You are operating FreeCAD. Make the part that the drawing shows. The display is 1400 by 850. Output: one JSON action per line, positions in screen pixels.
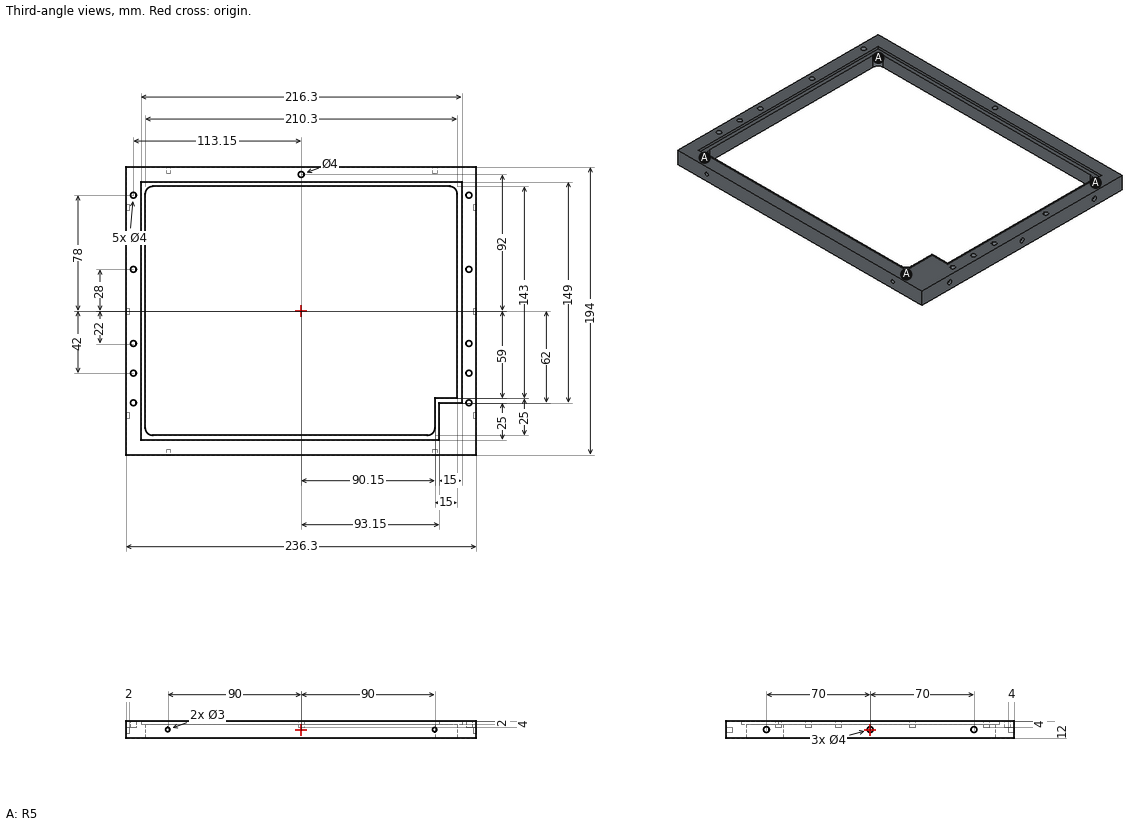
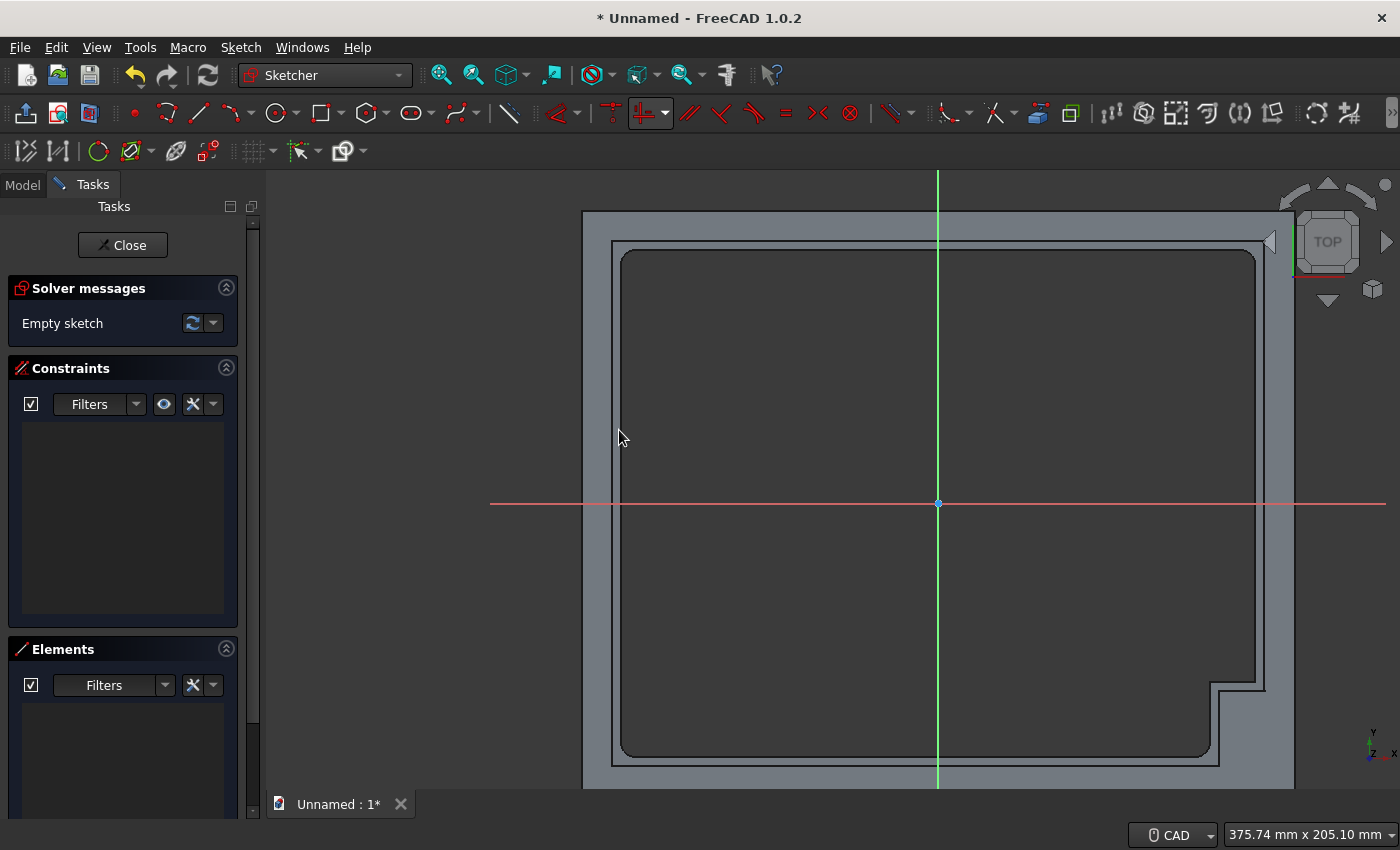
{"action": "left_click", "coordinate": [276, 114]}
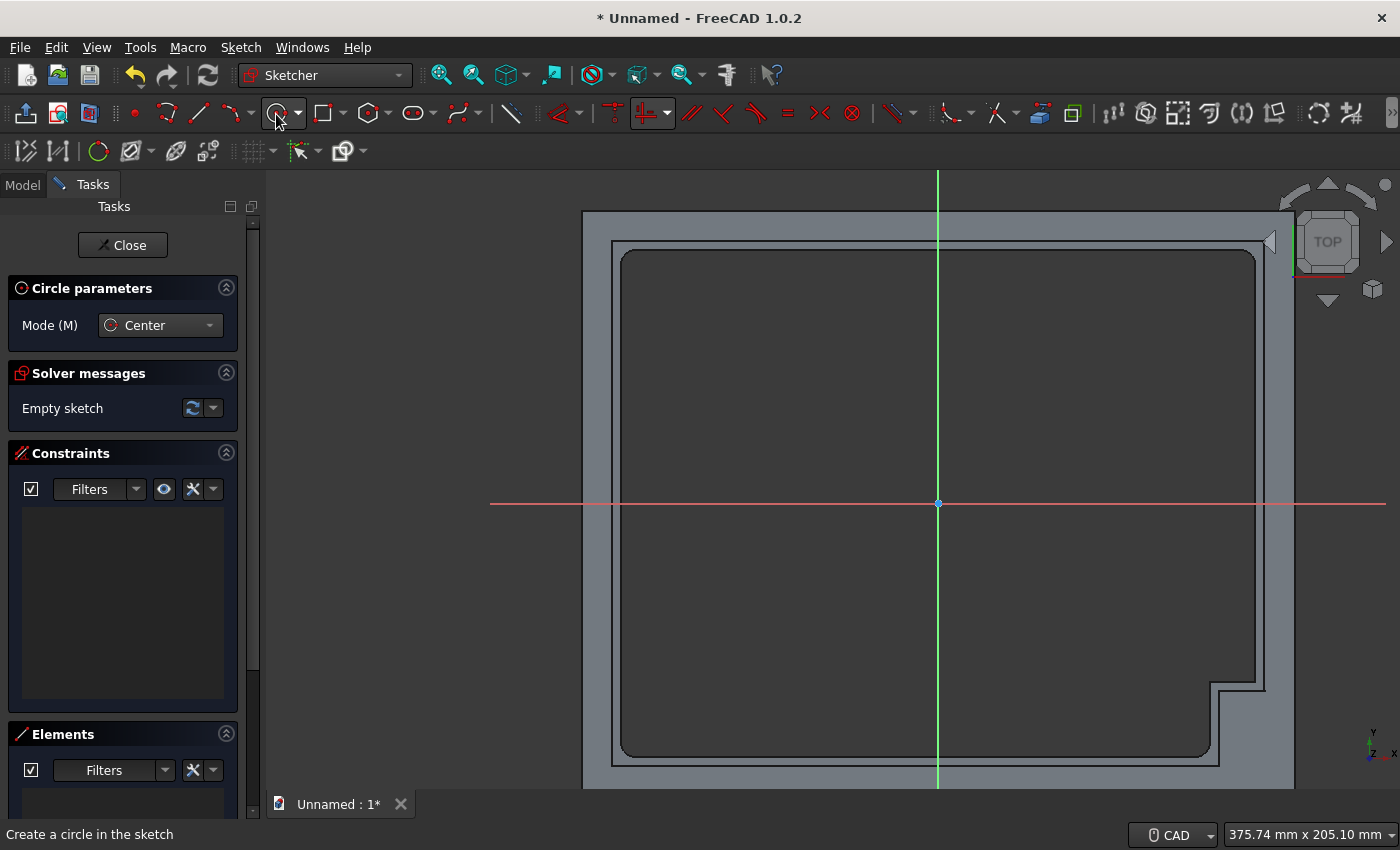
{"action": "scroll", "coordinate": [597, 268], "scroll_direction": "up", "scroll_amount": 7}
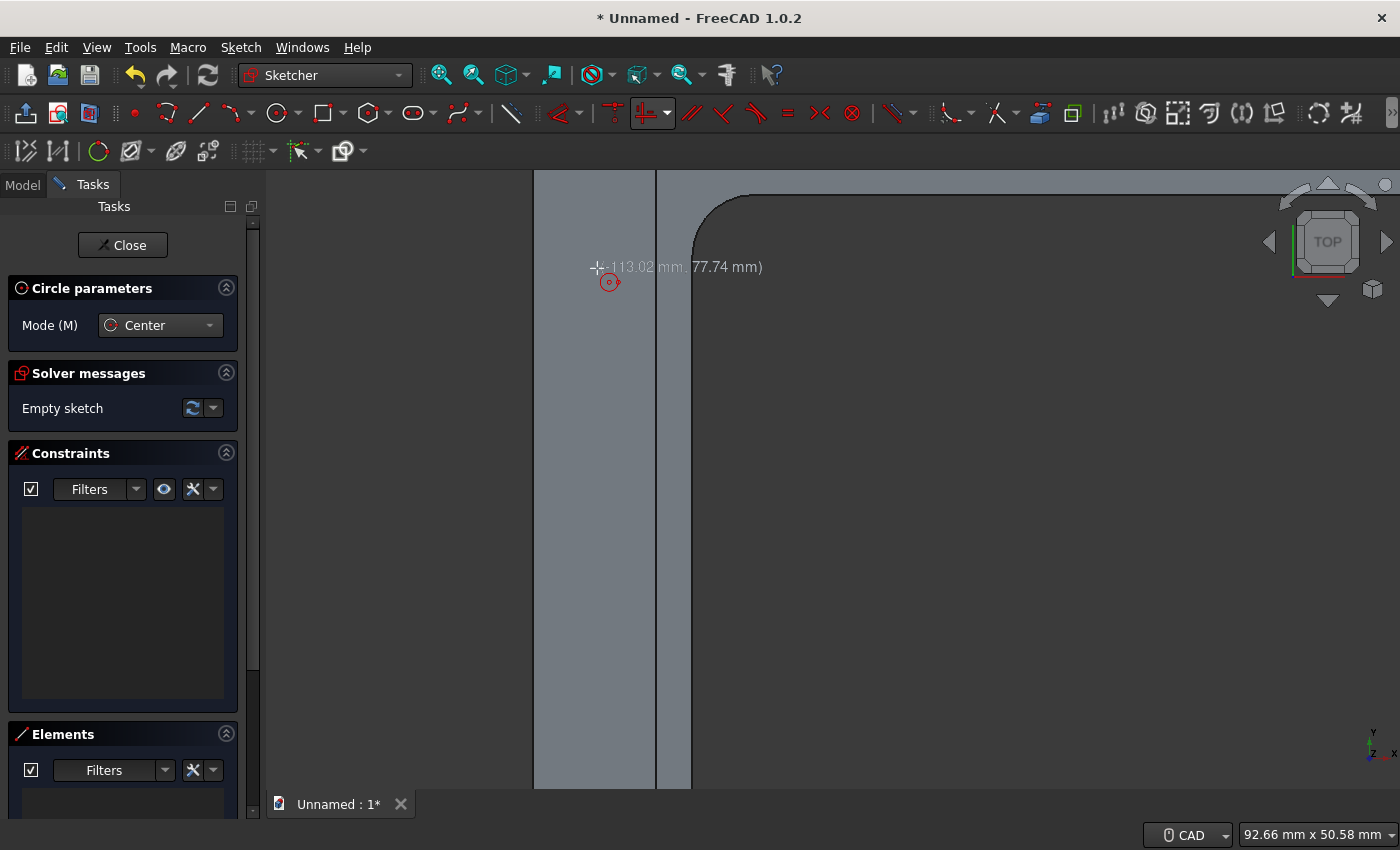
{"action": "scroll", "coordinate": [598, 268], "scroll_direction": "down", "scroll_amount": 7}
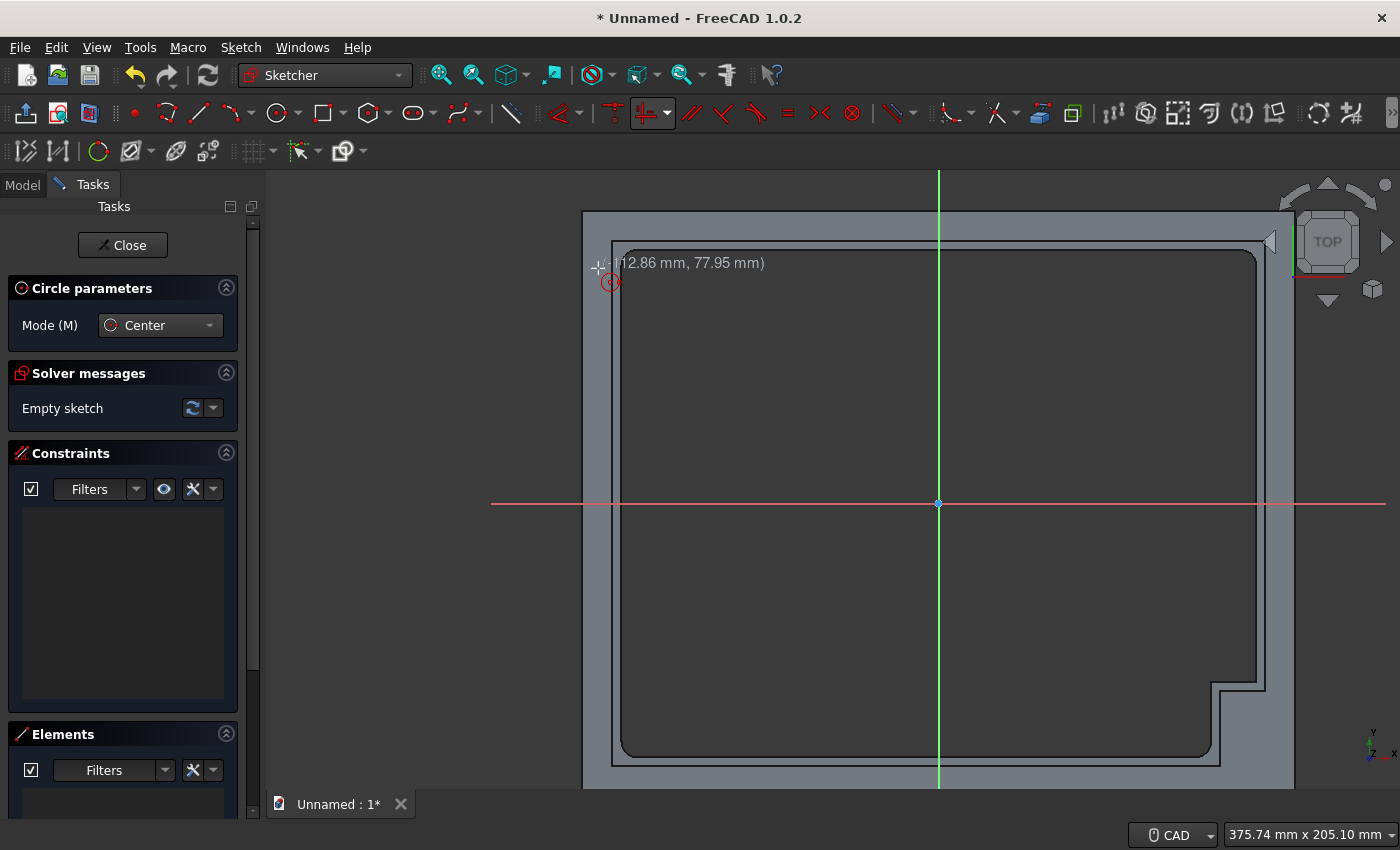
{"action": "left_click", "coordinate": [597, 268]}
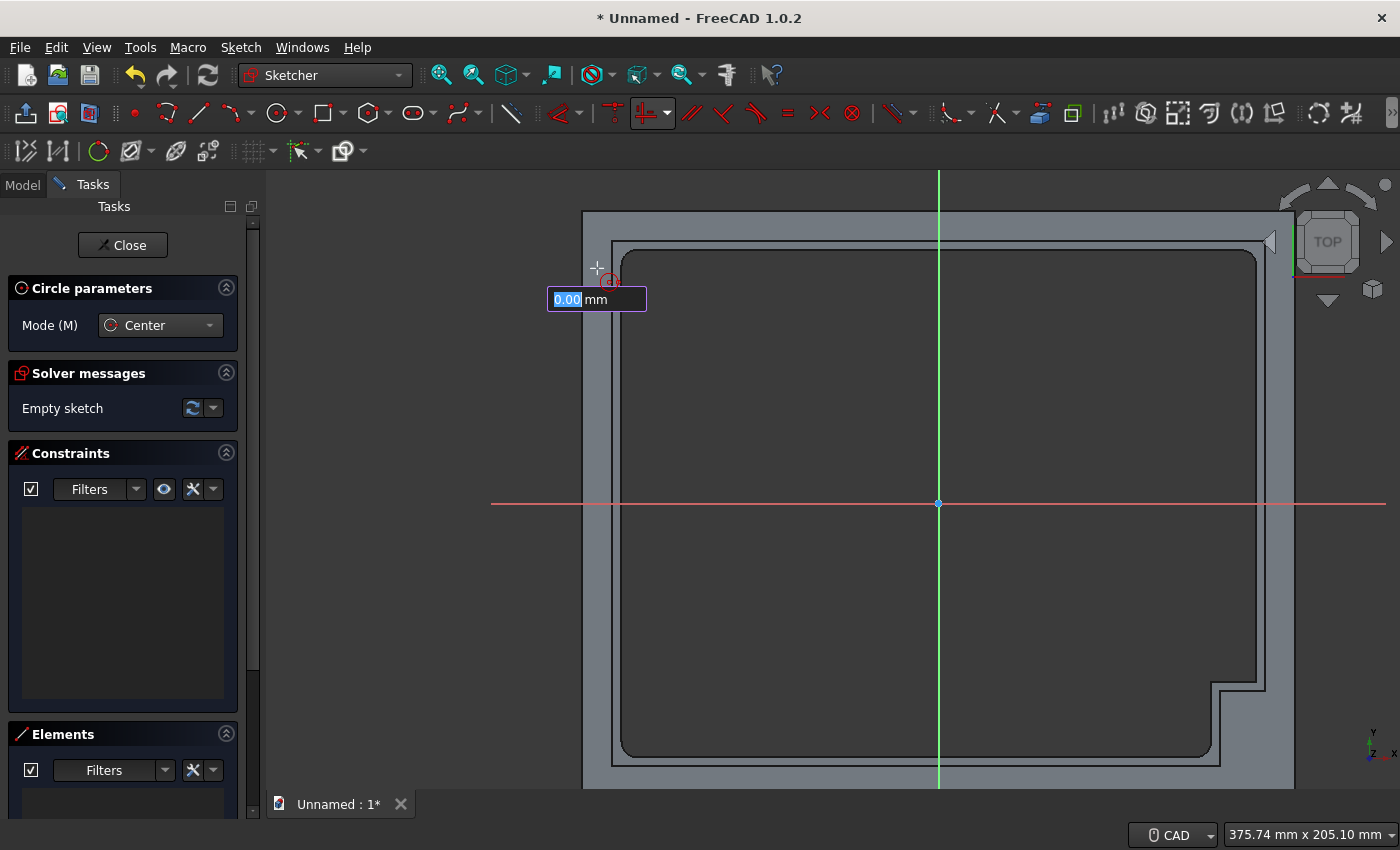
{"action": "scroll", "coordinate": [602, 264], "scroll_direction": "up", "scroll_amount": 5}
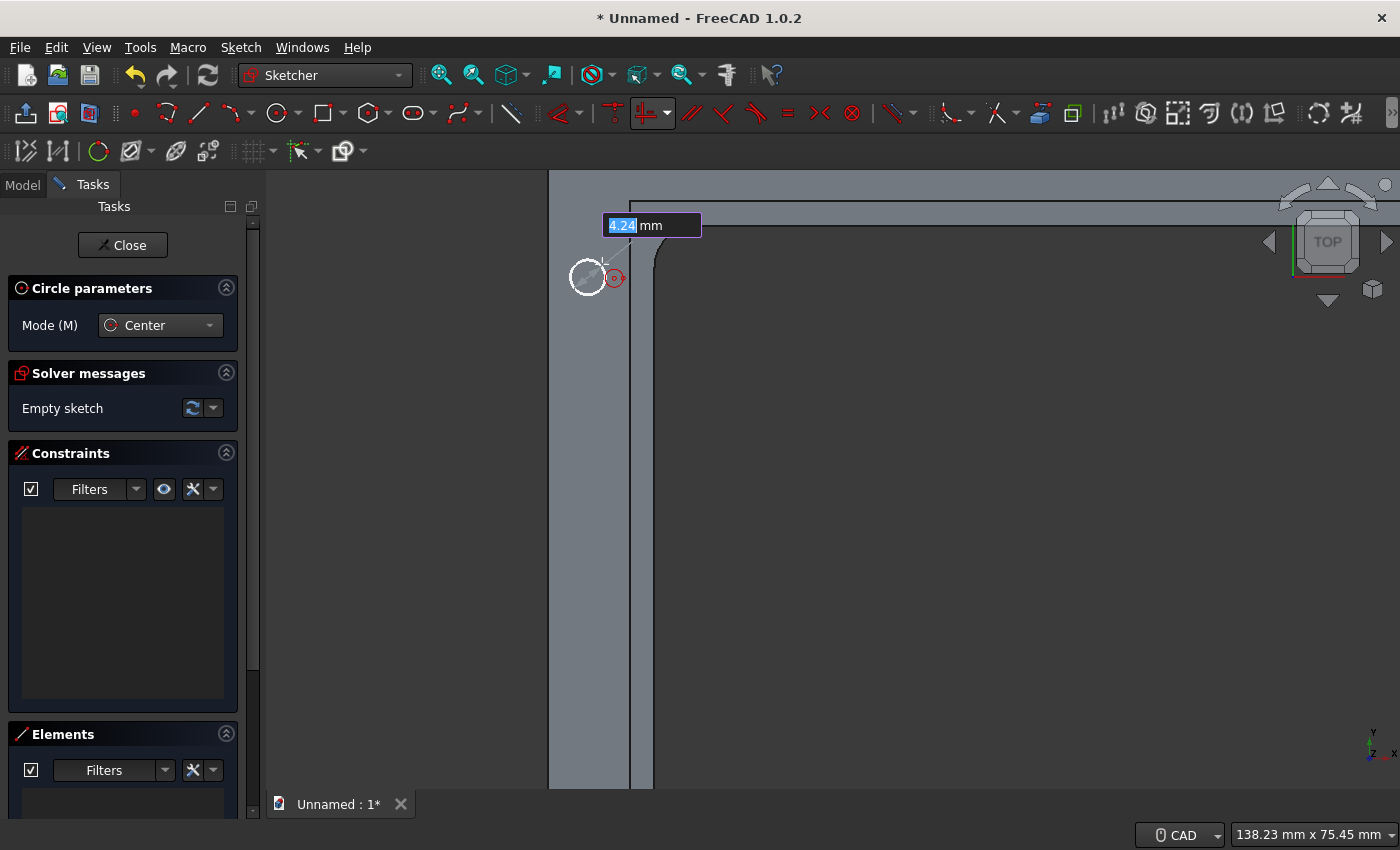
{"action": "left_click", "coordinate": [600, 264]}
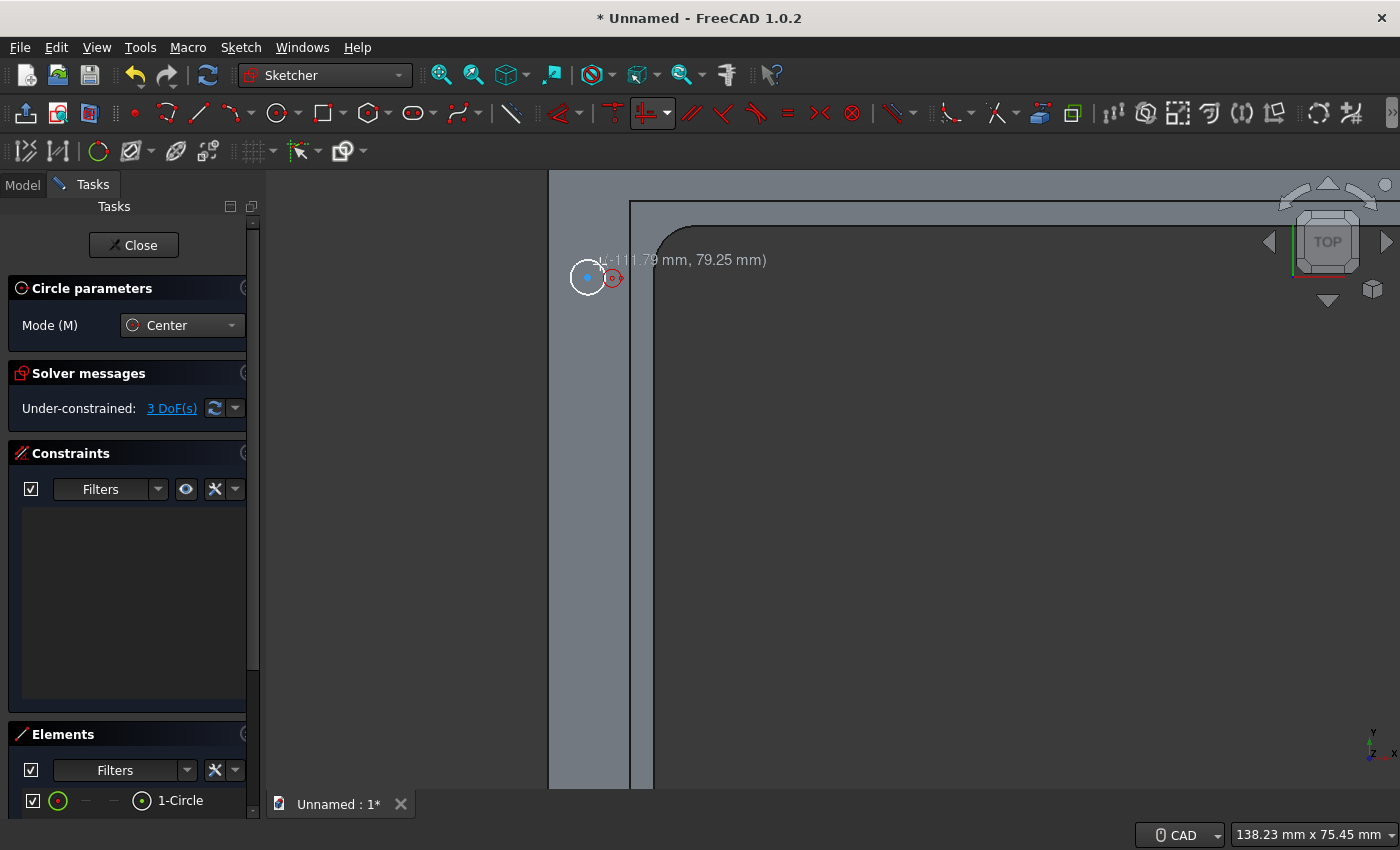
{"action": "scroll", "coordinate": [589, 685], "scroll_direction": "up", "scroll_amount": 2}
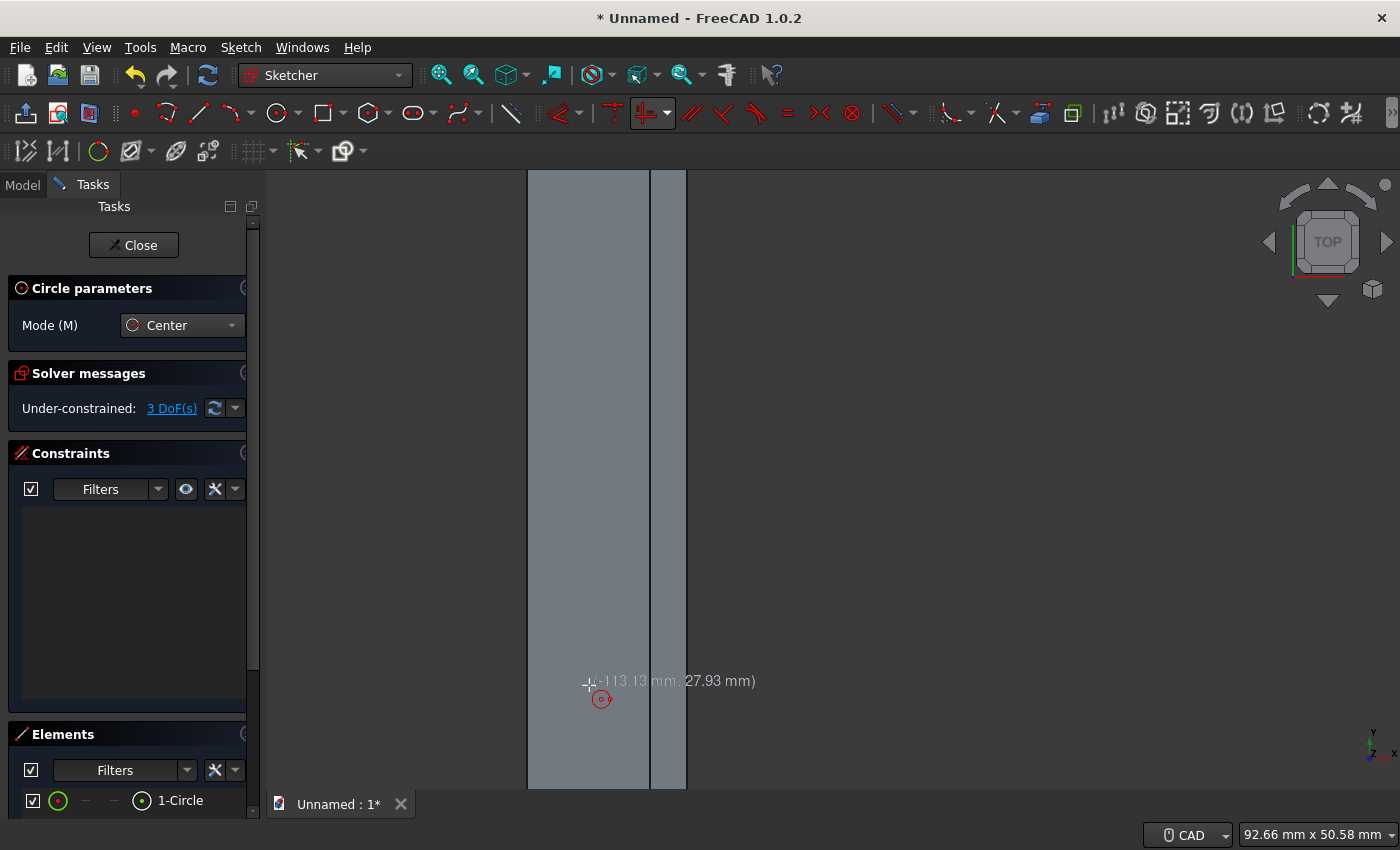
{"action": "scroll", "coordinate": [599, 332], "scroll_direction": "down", "scroll_amount": 7}